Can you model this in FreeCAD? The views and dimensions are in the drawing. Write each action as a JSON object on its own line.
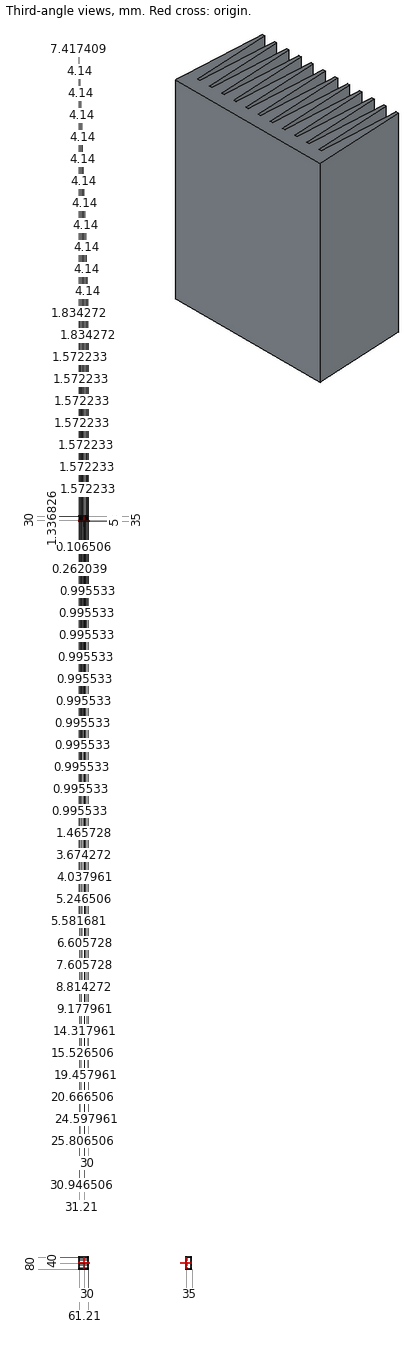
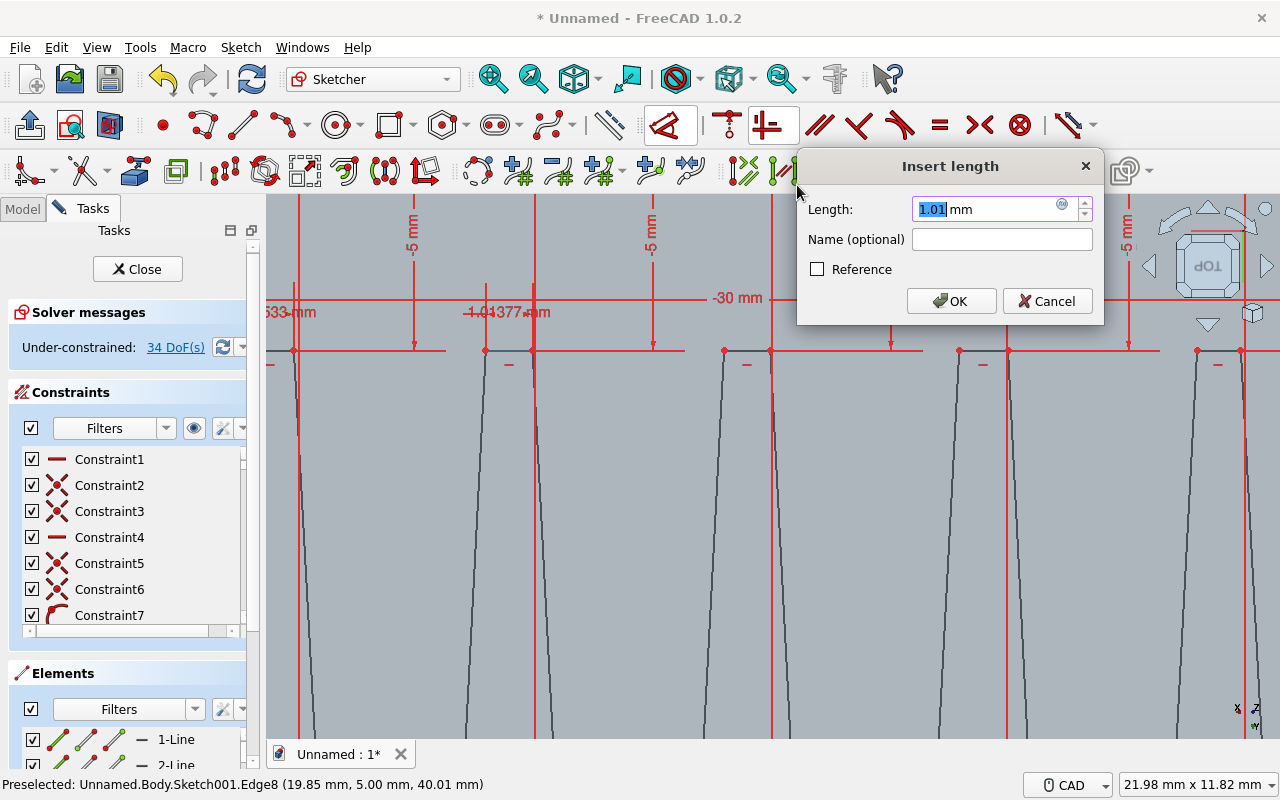
{"action": "type", "text": "0.995533"}
{"action": "key", "text": "Return"}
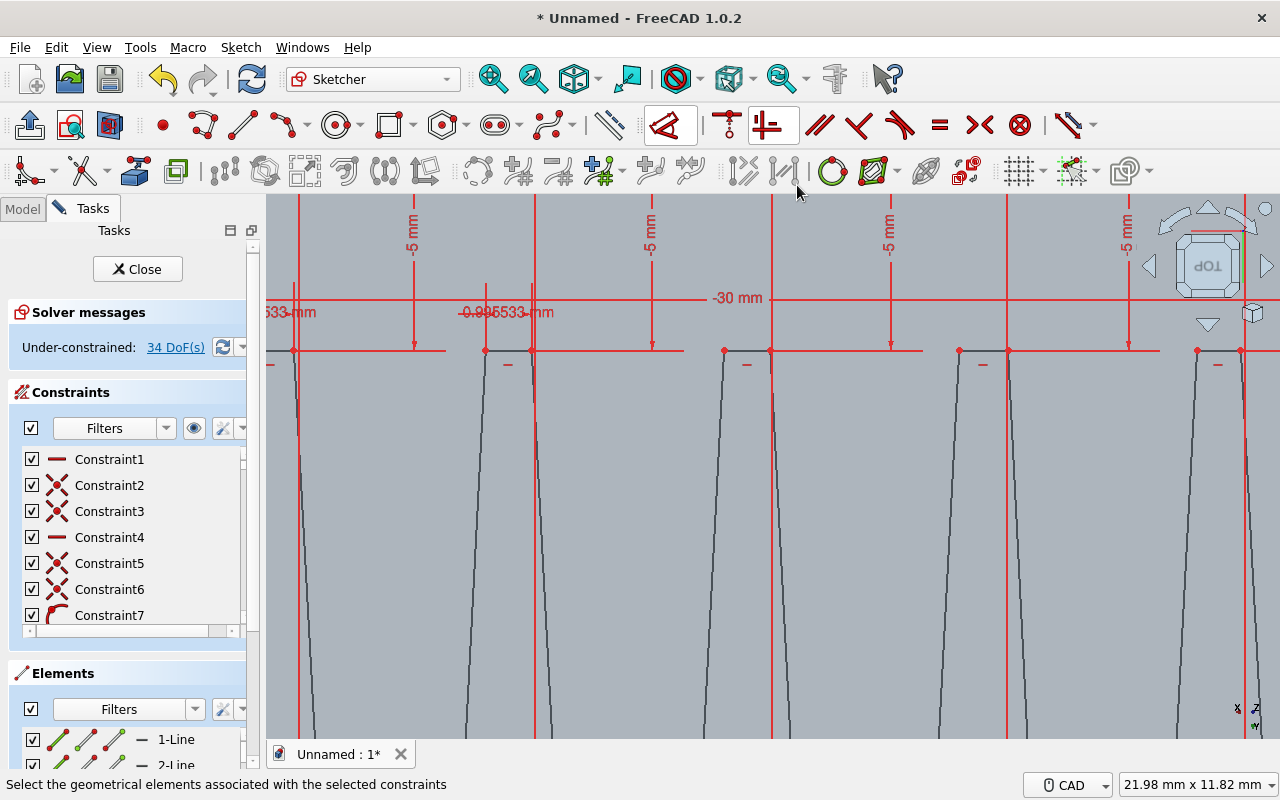
{"action": "left_click", "coordinate": [756, 351]}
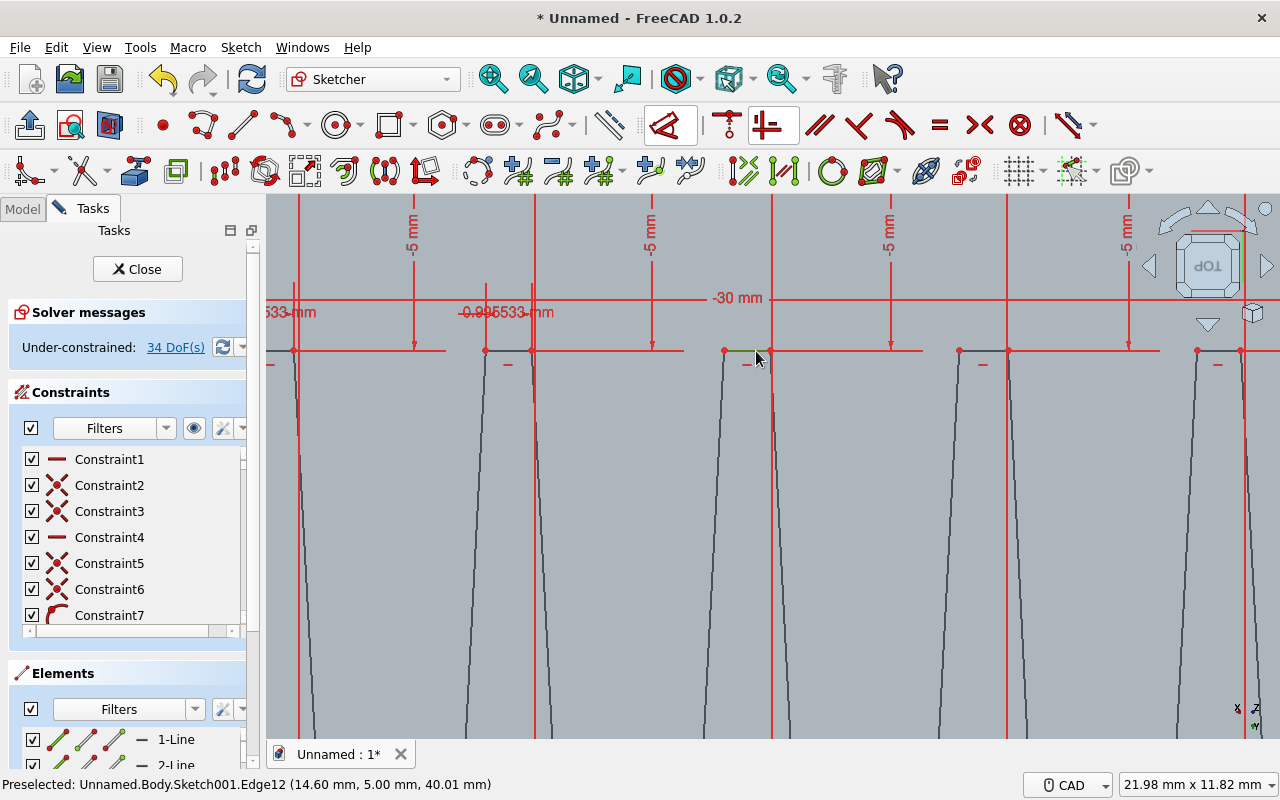
{"action": "left_click", "coordinate": [692, 126]}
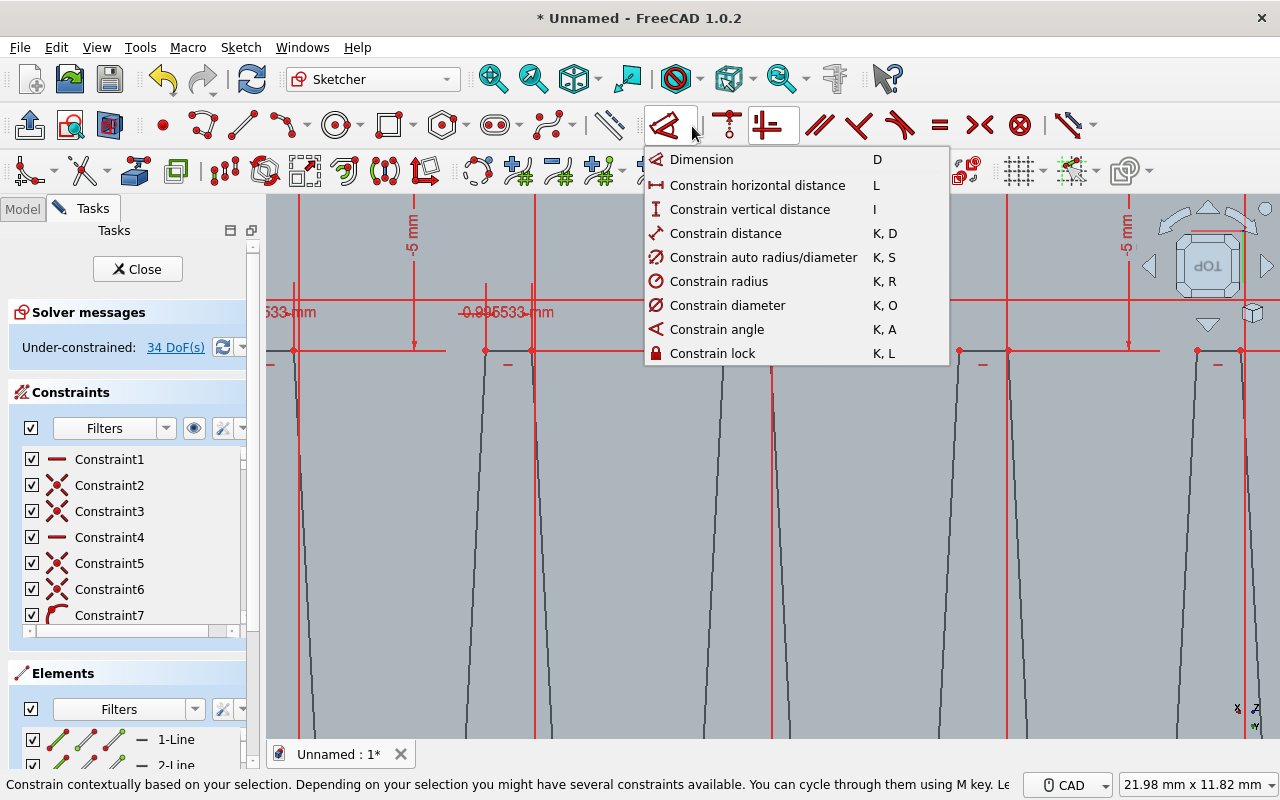
{"action": "left_click", "coordinate": [797, 185]}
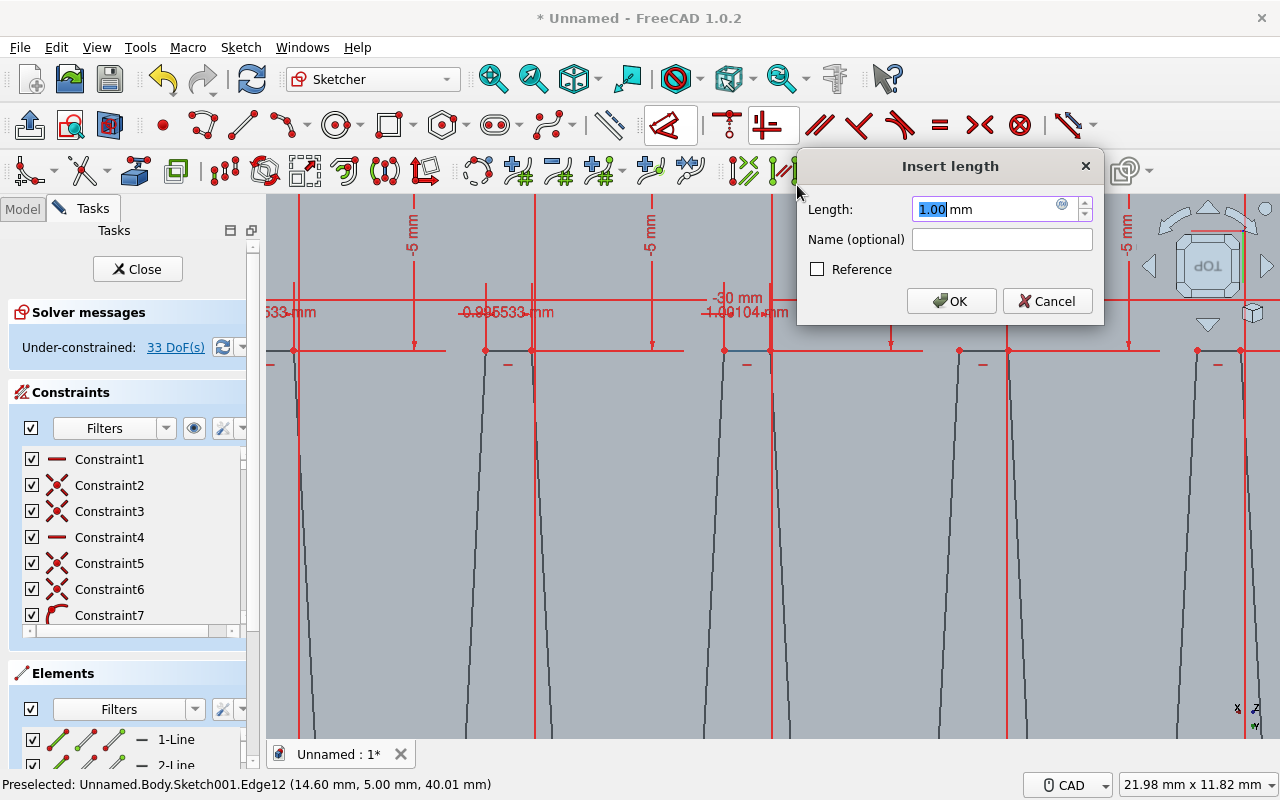
{"action": "type", "text": "0.995533"}
{"action": "key", "text": "Return"}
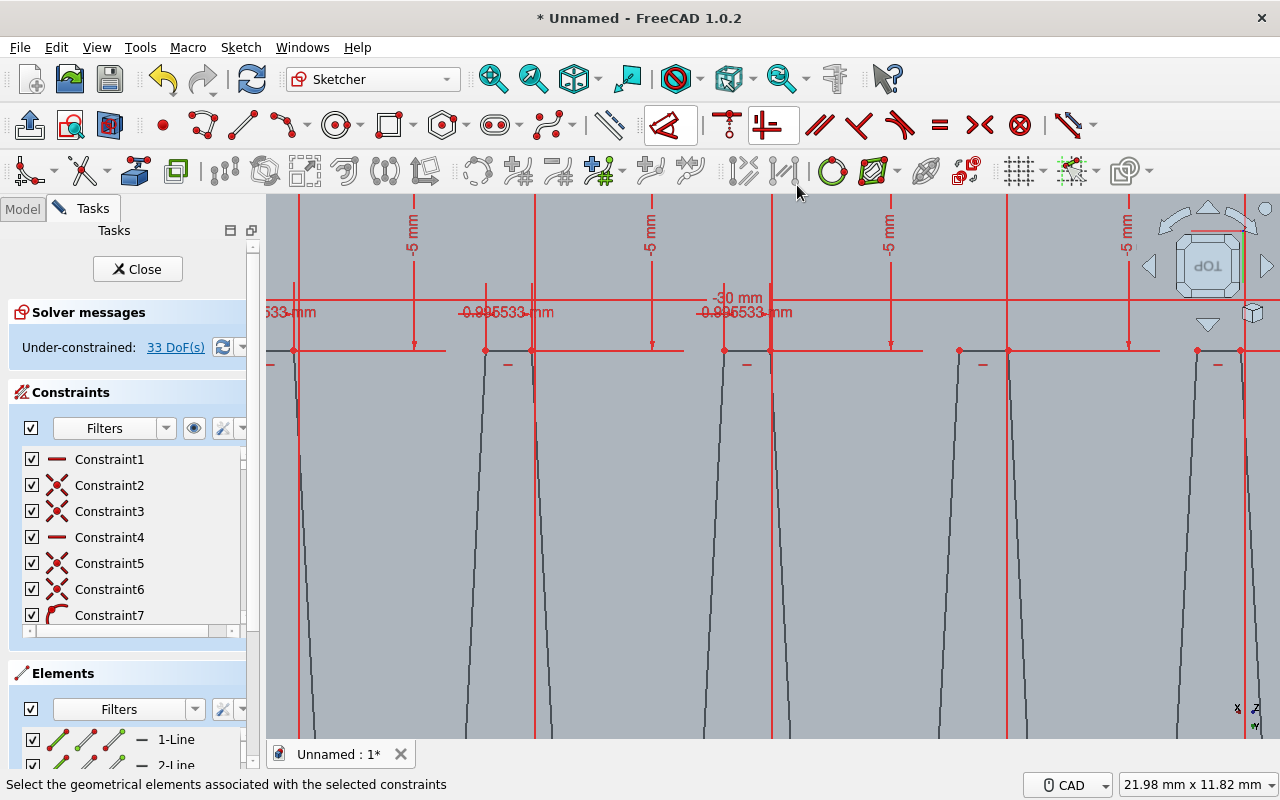
{"action": "left_click", "coordinate": [993, 351]}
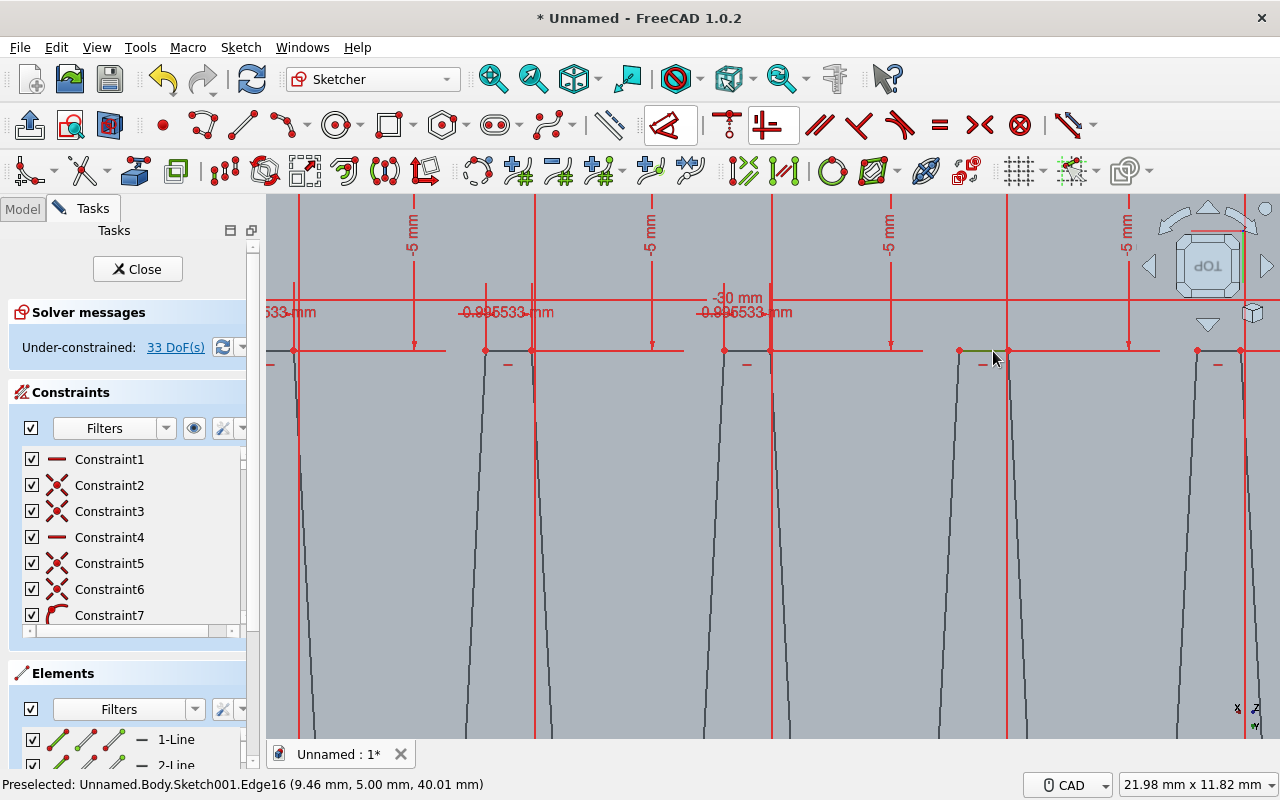
{"action": "left_click", "coordinate": [692, 126]}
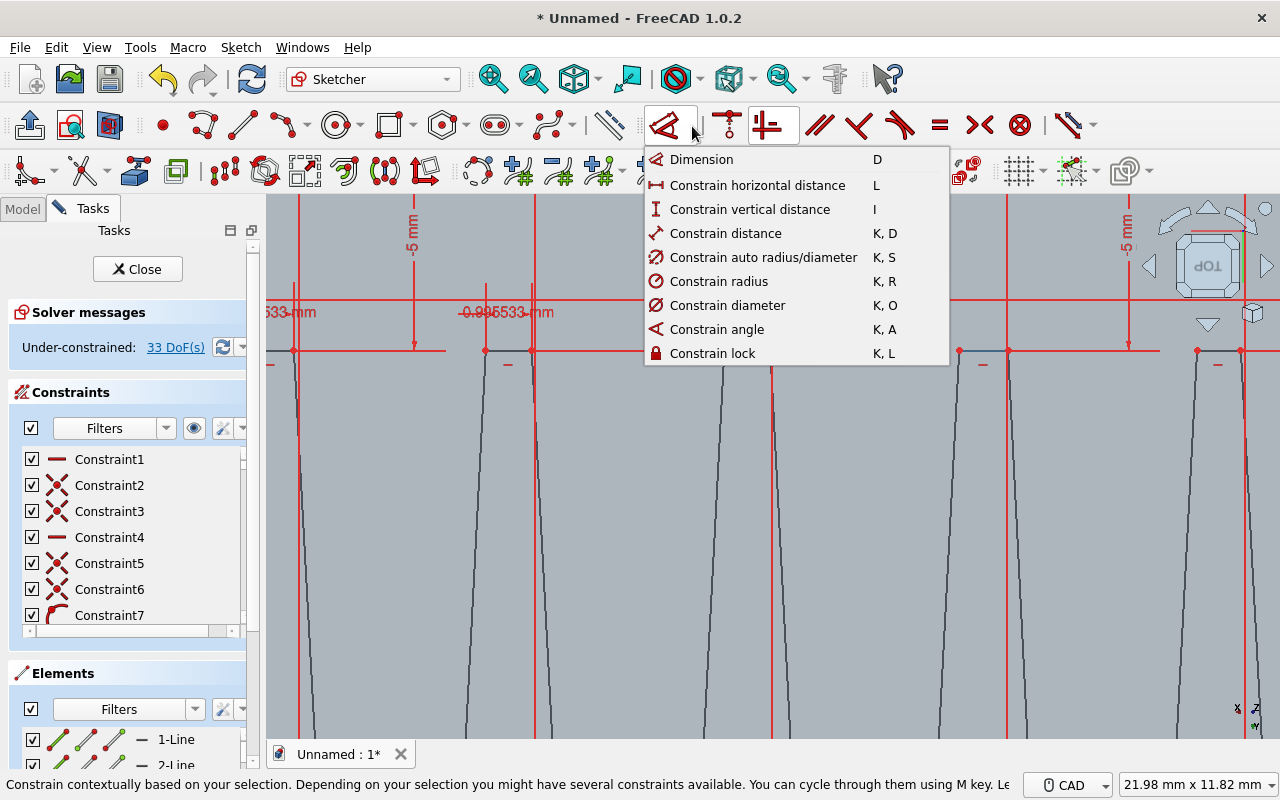
{"action": "left_click", "coordinate": [797, 185]}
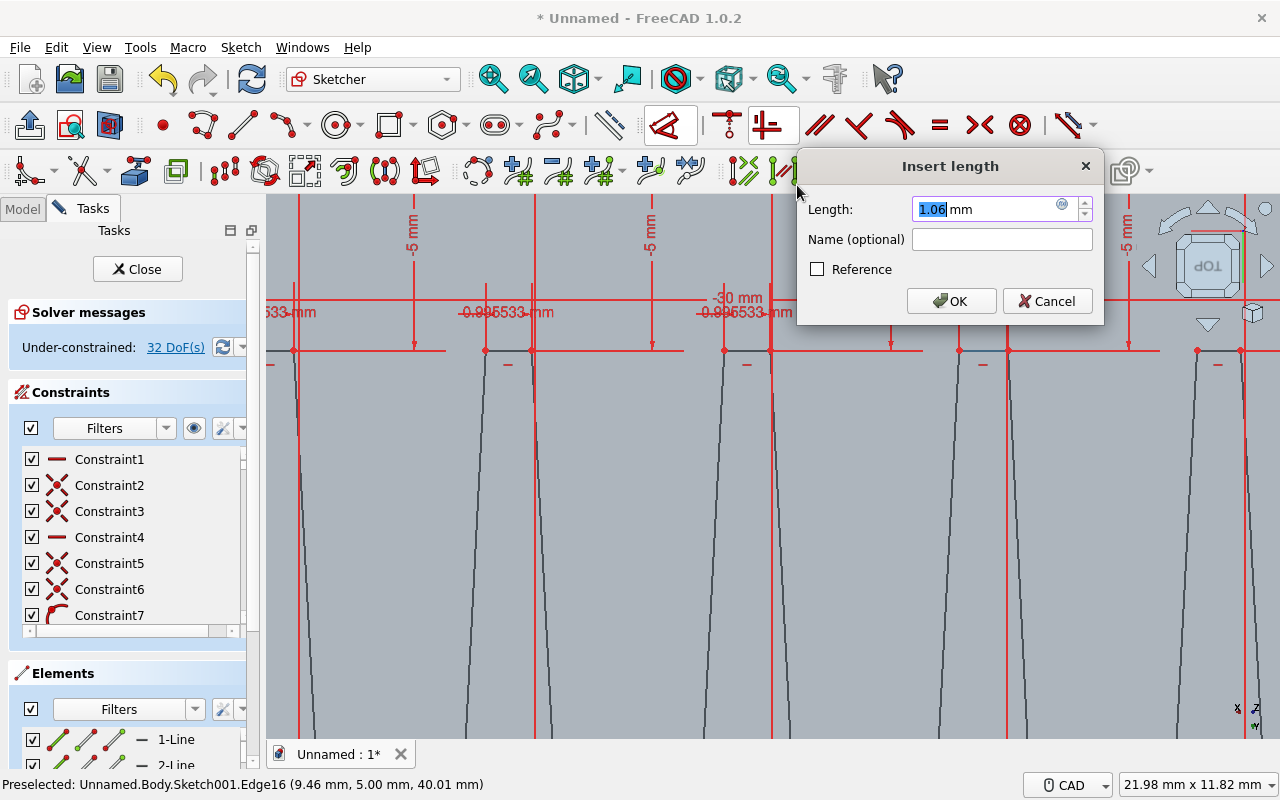
{"action": "type", "text": "0.995533"}
{"action": "key", "text": "Return"}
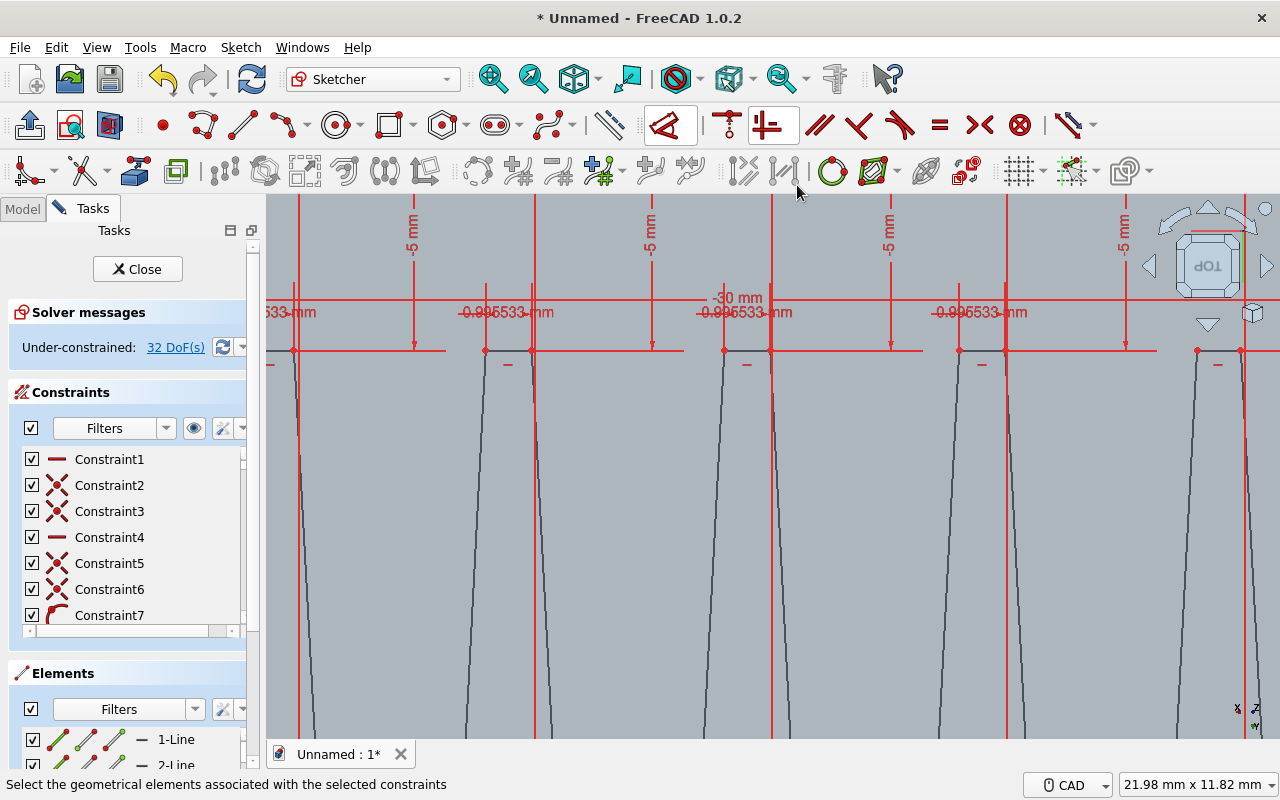
{"action": "scroll", "coordinate": [514, 350], "scroll_direction": "down", "scroll_amount": 8}